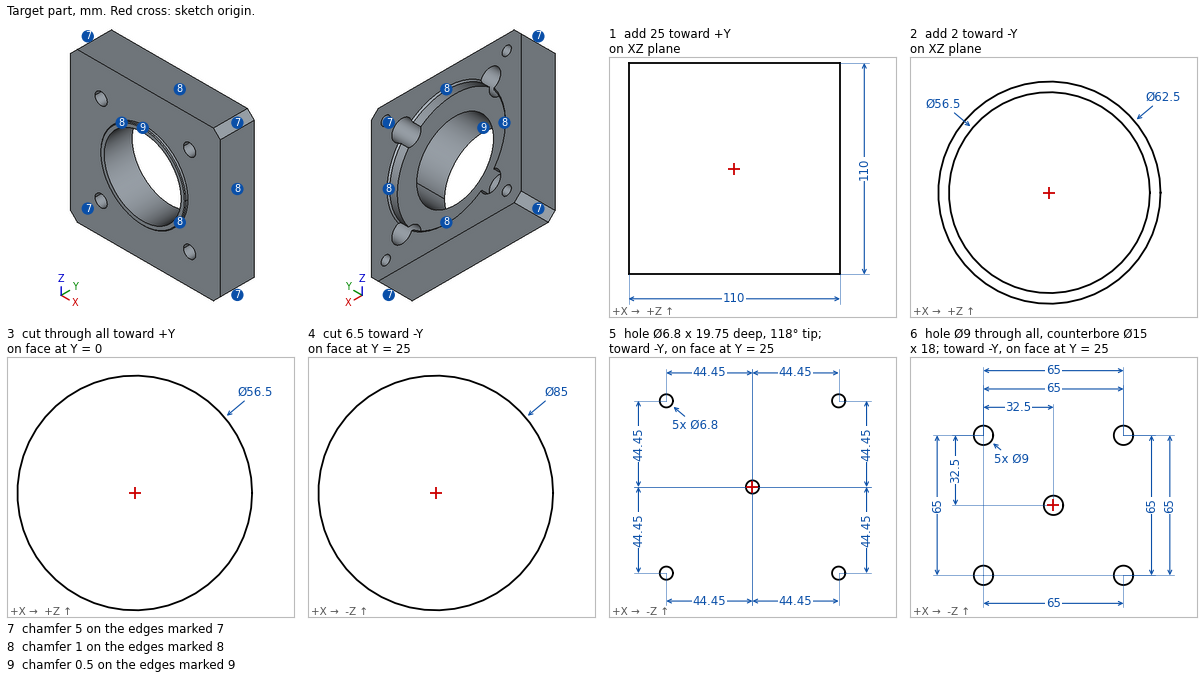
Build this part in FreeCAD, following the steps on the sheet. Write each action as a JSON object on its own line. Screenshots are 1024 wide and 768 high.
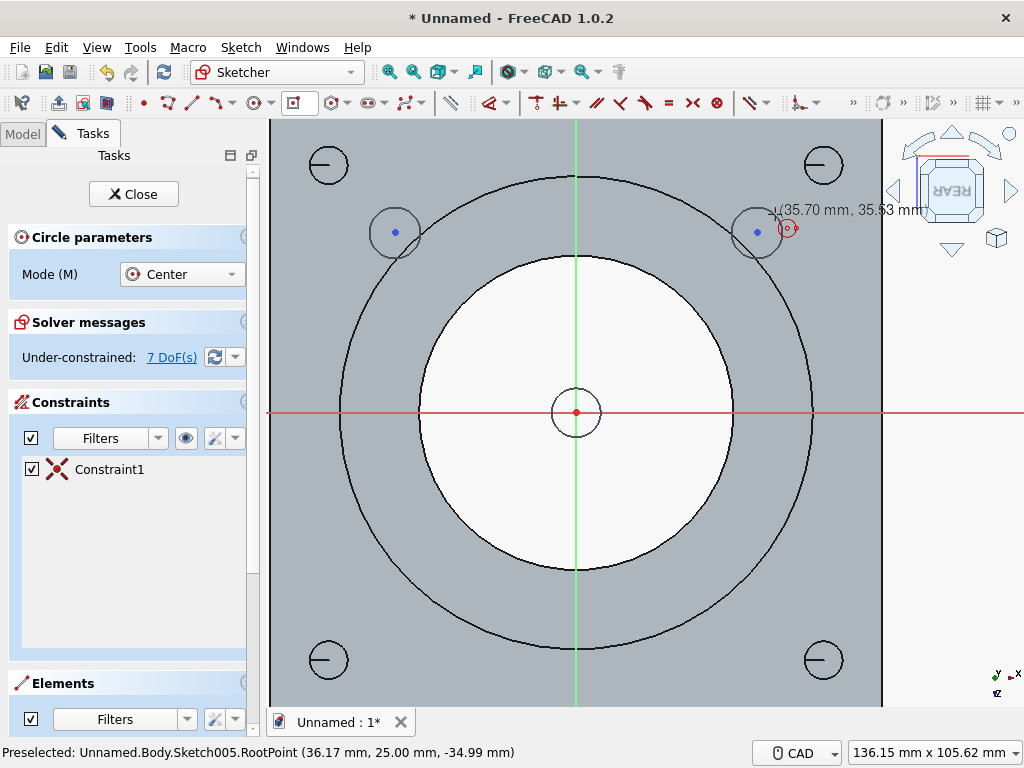
{"action": "left_click", "coordinate": [395, 594]}
{"action": "left_click", "coordinate": [413, 576]}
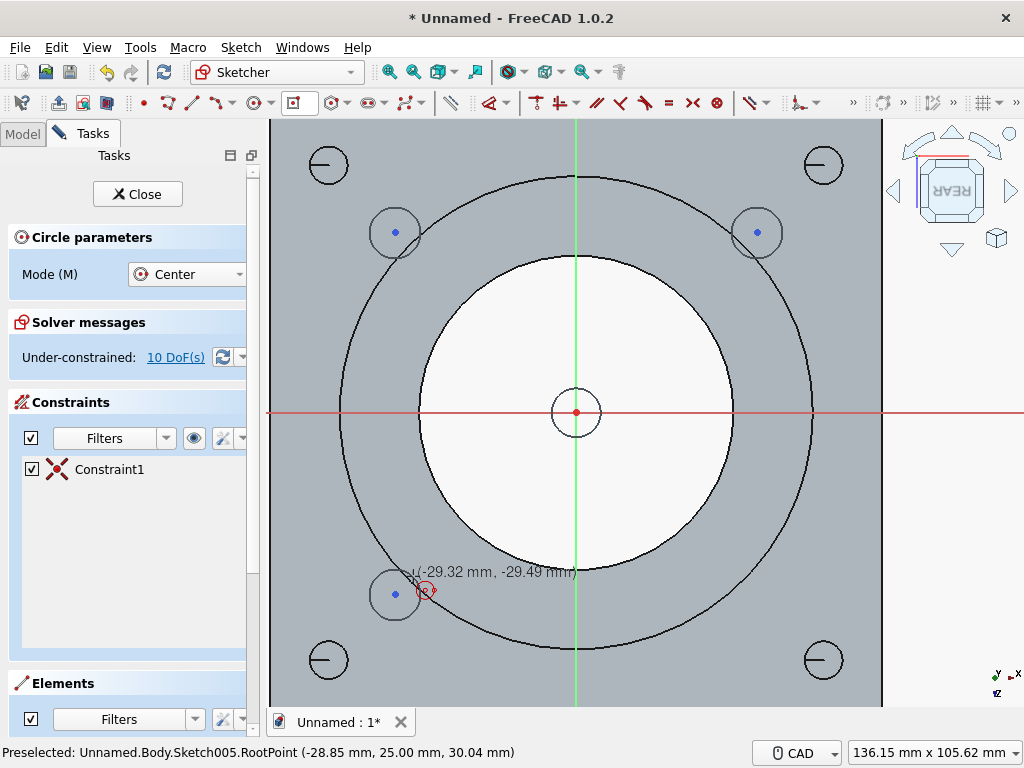
{"action": "left_click", "coordinate": [757, 594]}
{"action": "left_click", "coordinate": [775, 576]}
{"action": "key", "text": "Escape"}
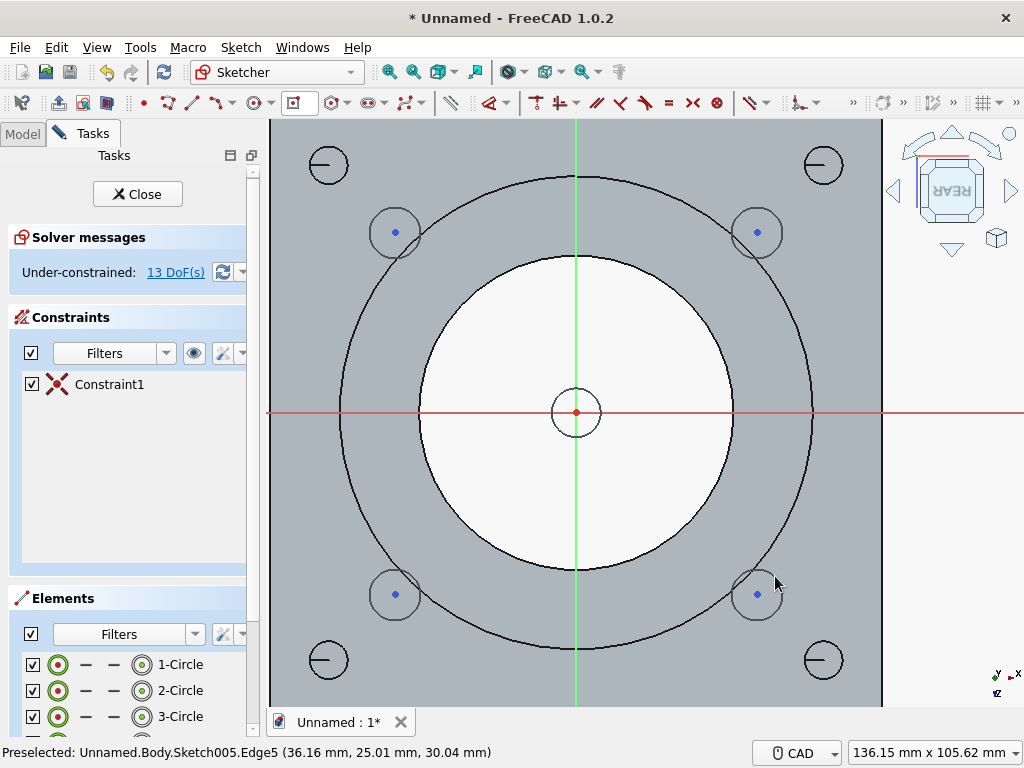
{"action": "left_click", "coordinate": [413, 215]}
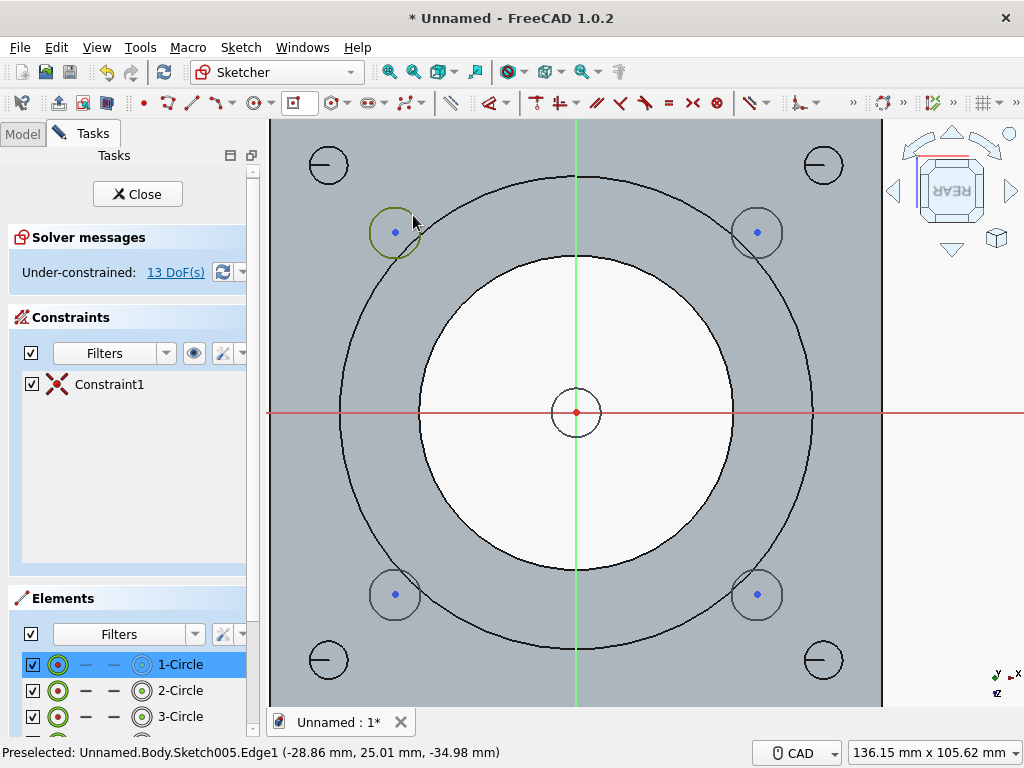
{"action": "left_click", "coordinate": [593, 395]}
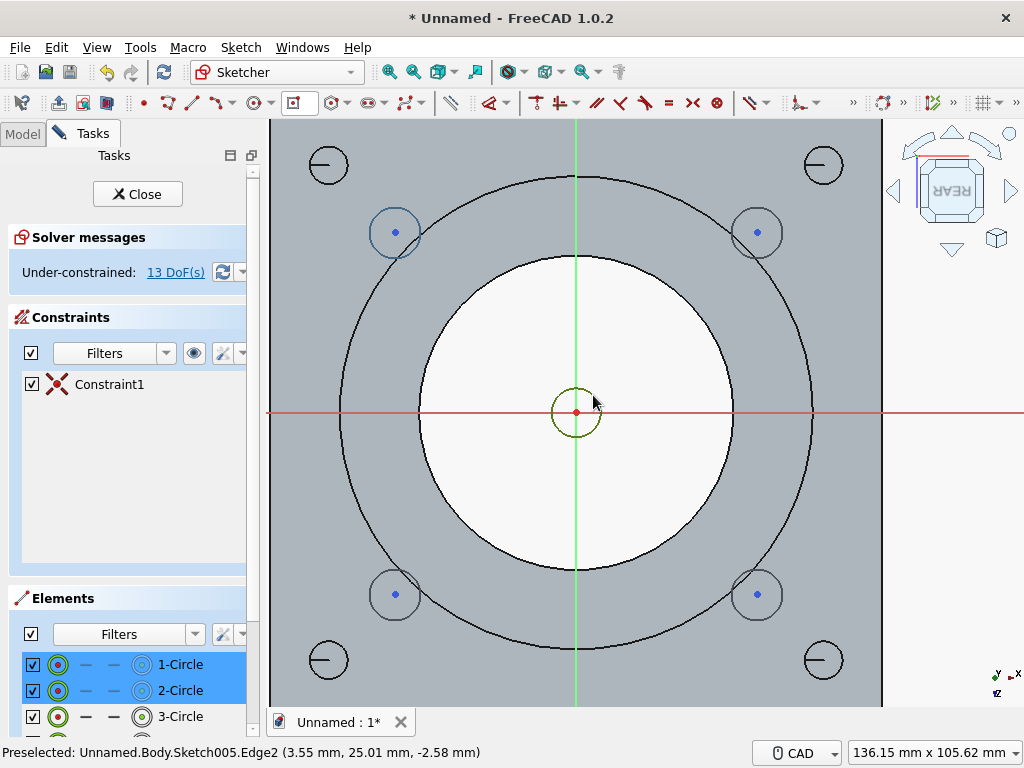
{"action": "left_click", "coordinate": [775, 215]}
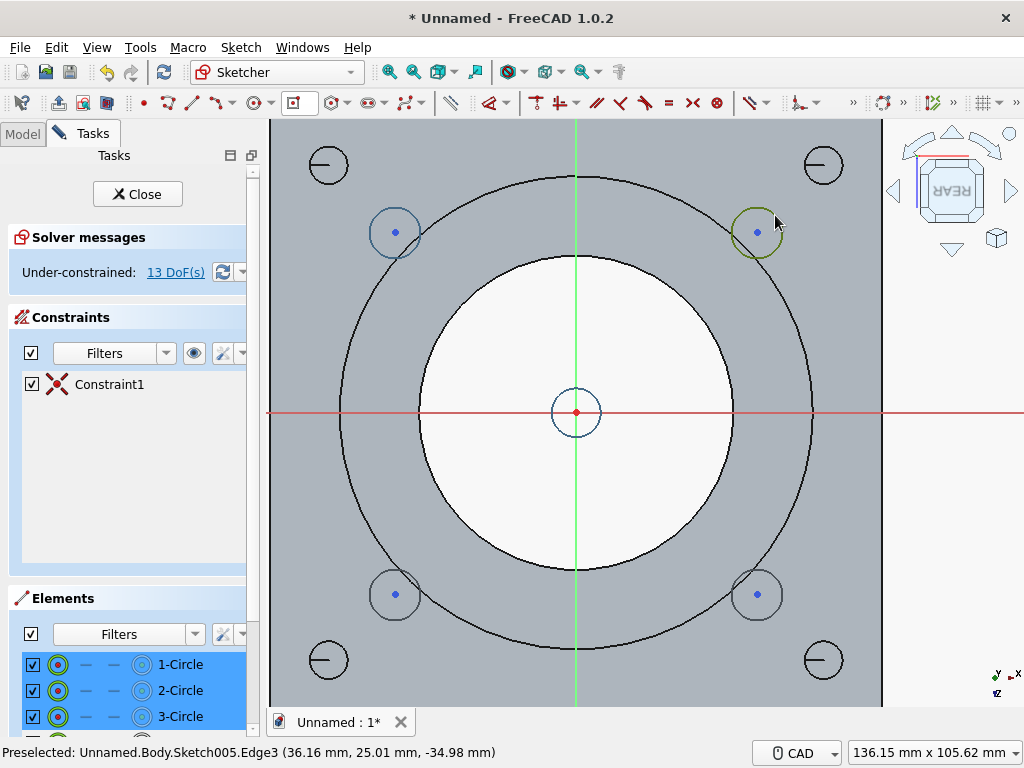
{"action": "left_click", "coordinate": [413, 577]}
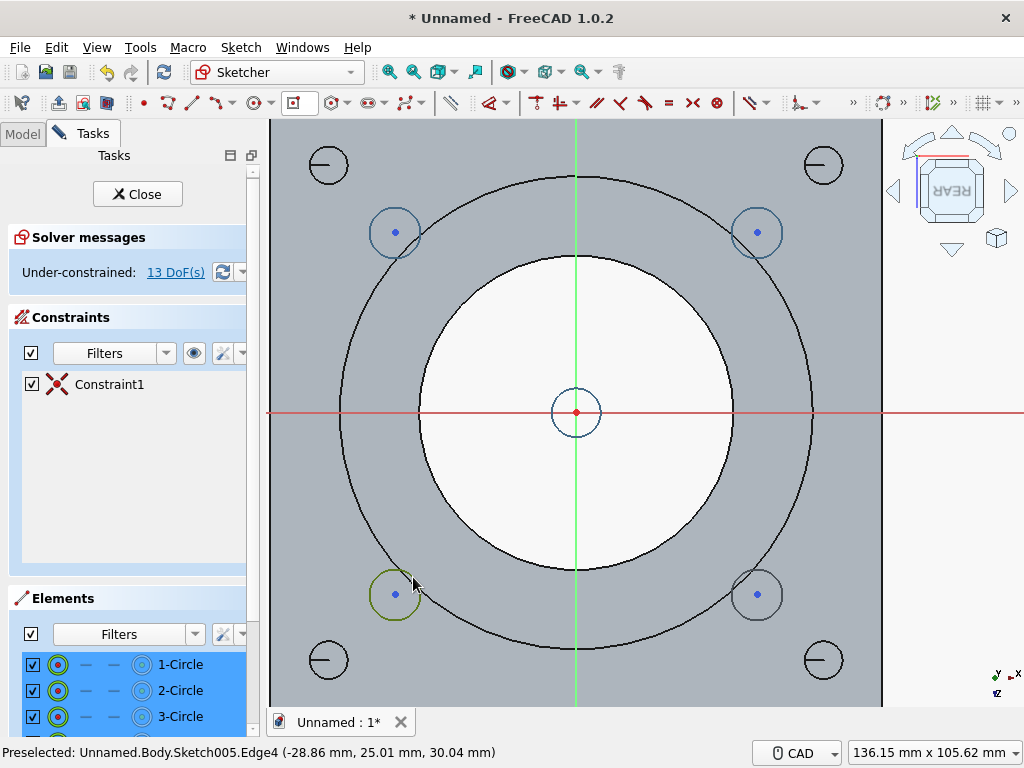
{"action": "left_click", "coordinate": [775, 577]}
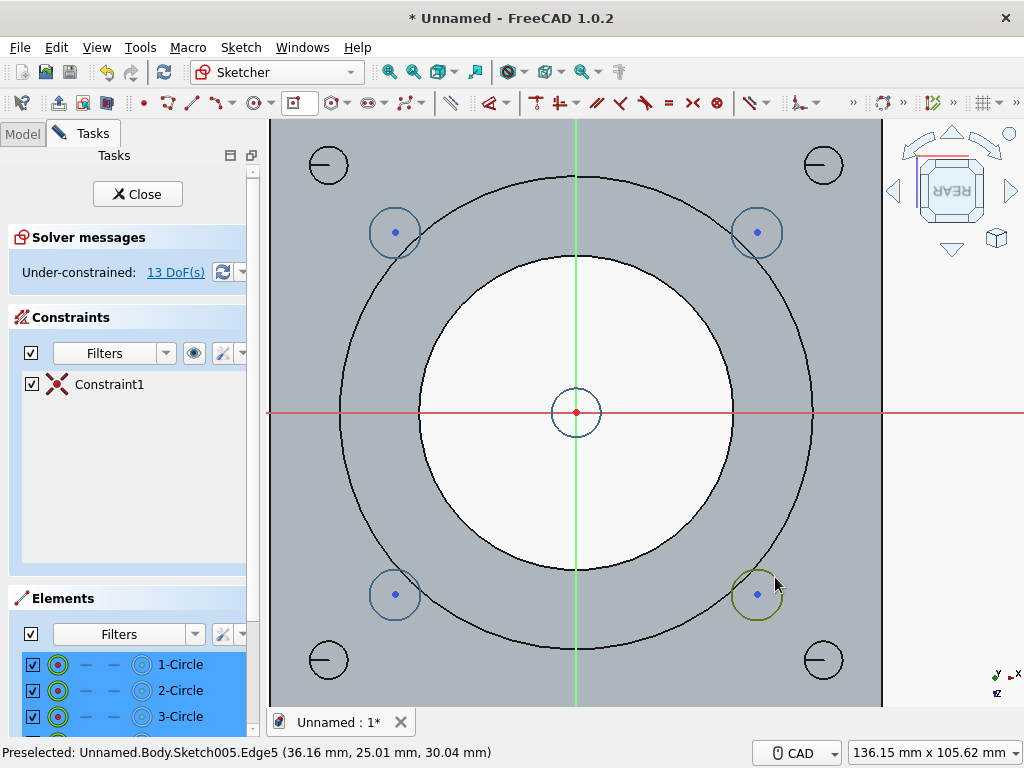
{"action": "left_click", "coordinate": [670, 104]}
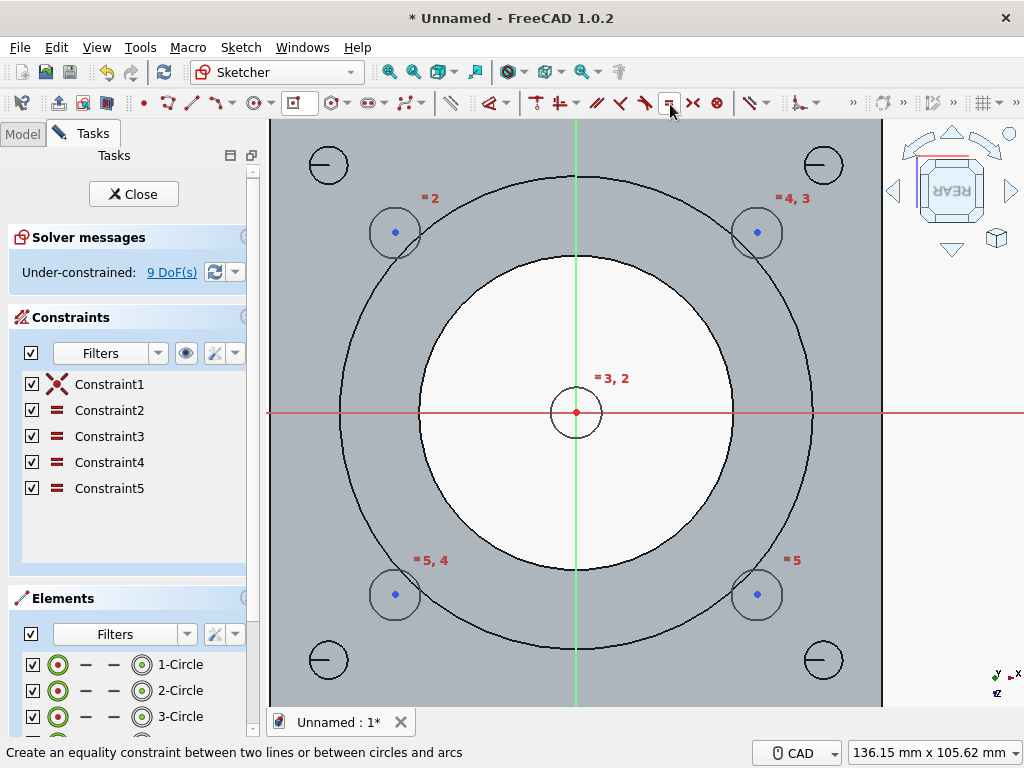
{"action": "left_click", "coordinate": [490, 104]}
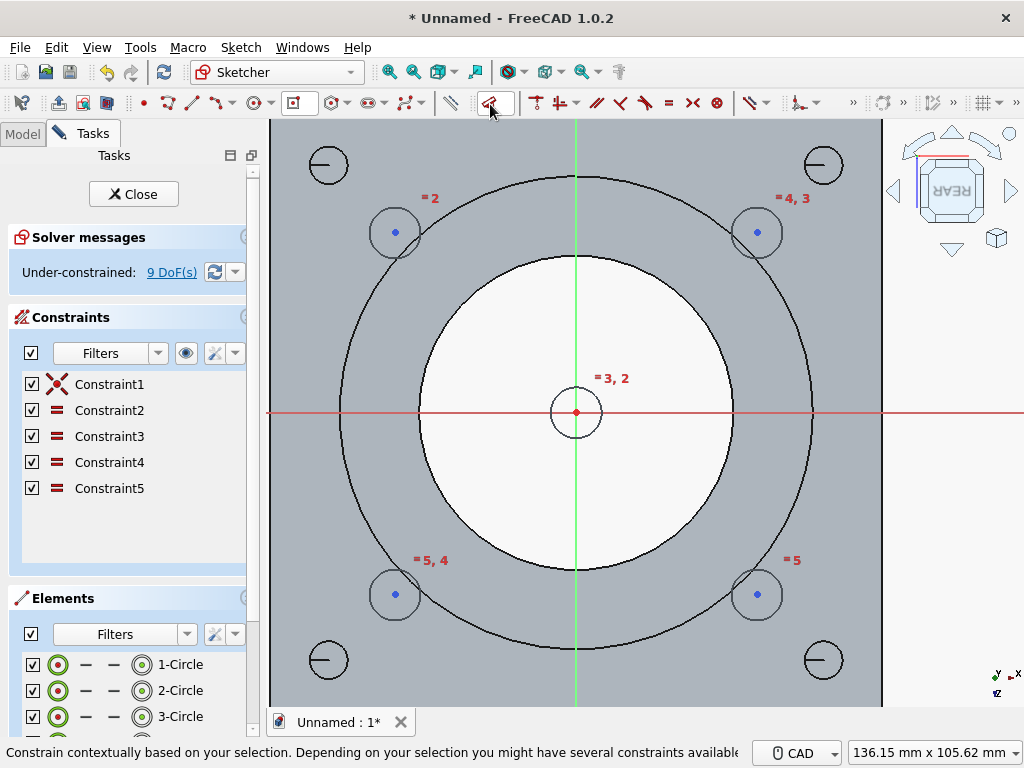
{"action": "left_click", "coordinate": [413, 215]}
{"action": "left_click", "coordinate": [436, 192]}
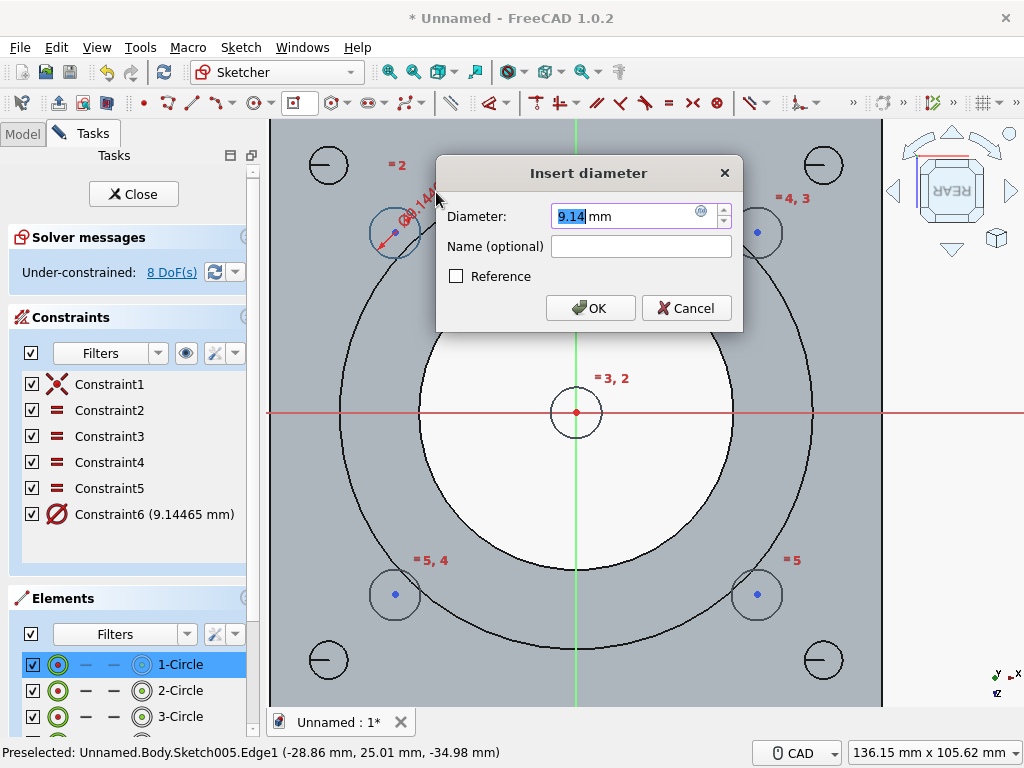
{"action": "type", "text": "9"}
{"action": "key", "text": "Return"}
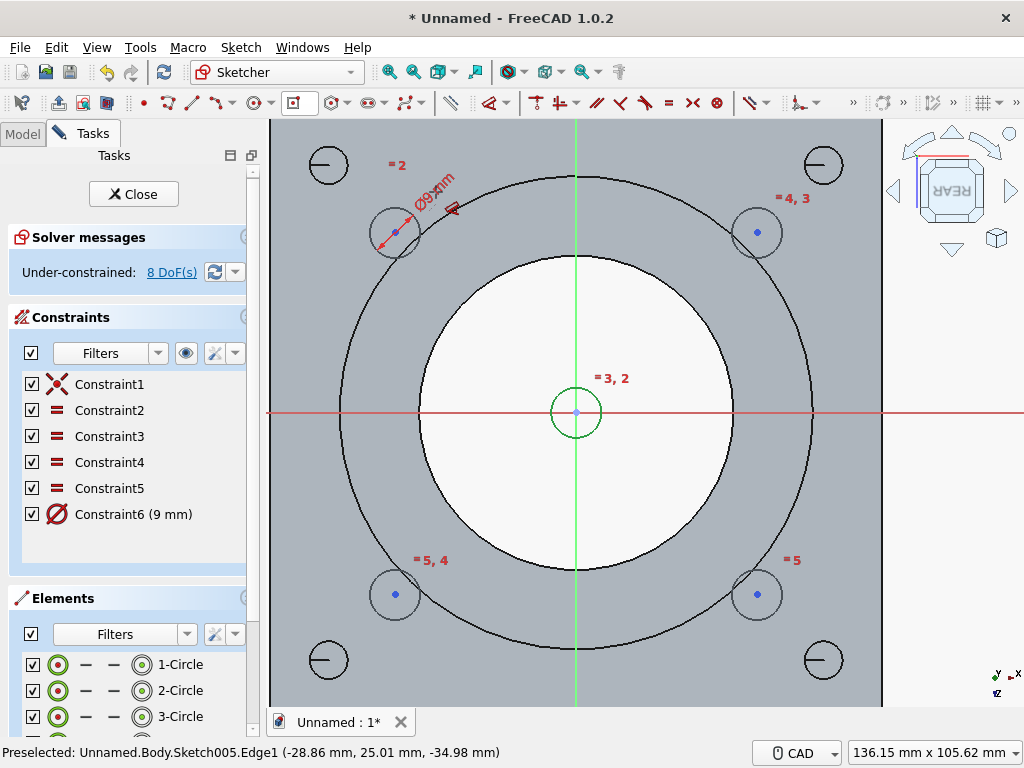
{"action": "left_click", "coordinate": [395, 233]}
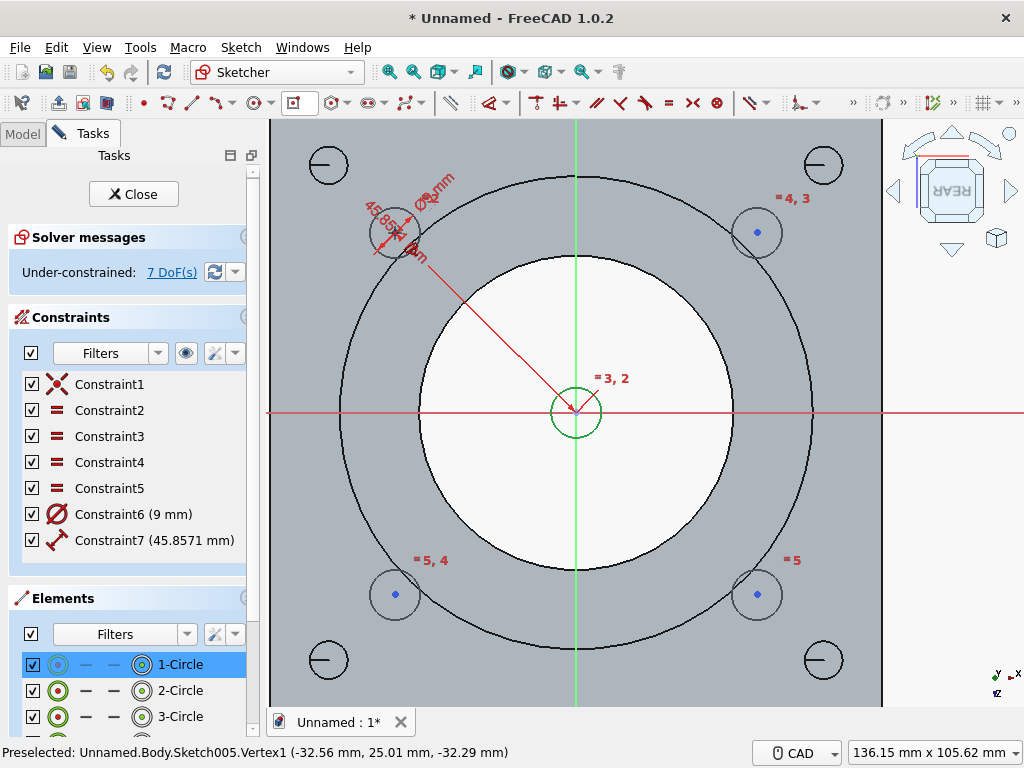
{"action": "left_click", "coordinate": [757, 233]}
{"action": "left_click", "coordinate": [659, 199]}